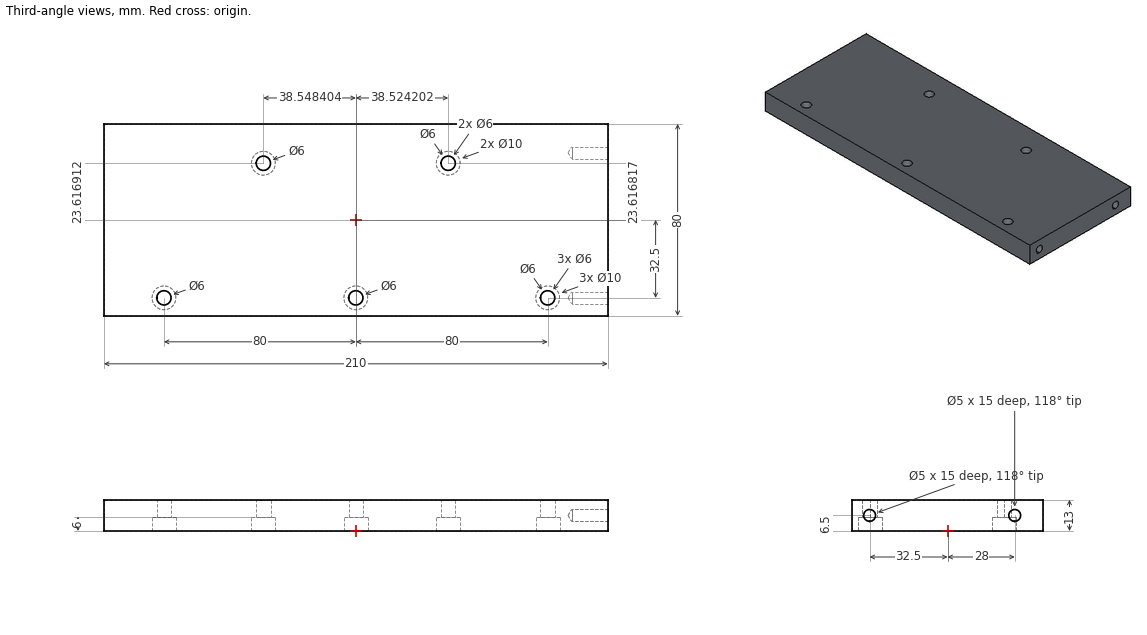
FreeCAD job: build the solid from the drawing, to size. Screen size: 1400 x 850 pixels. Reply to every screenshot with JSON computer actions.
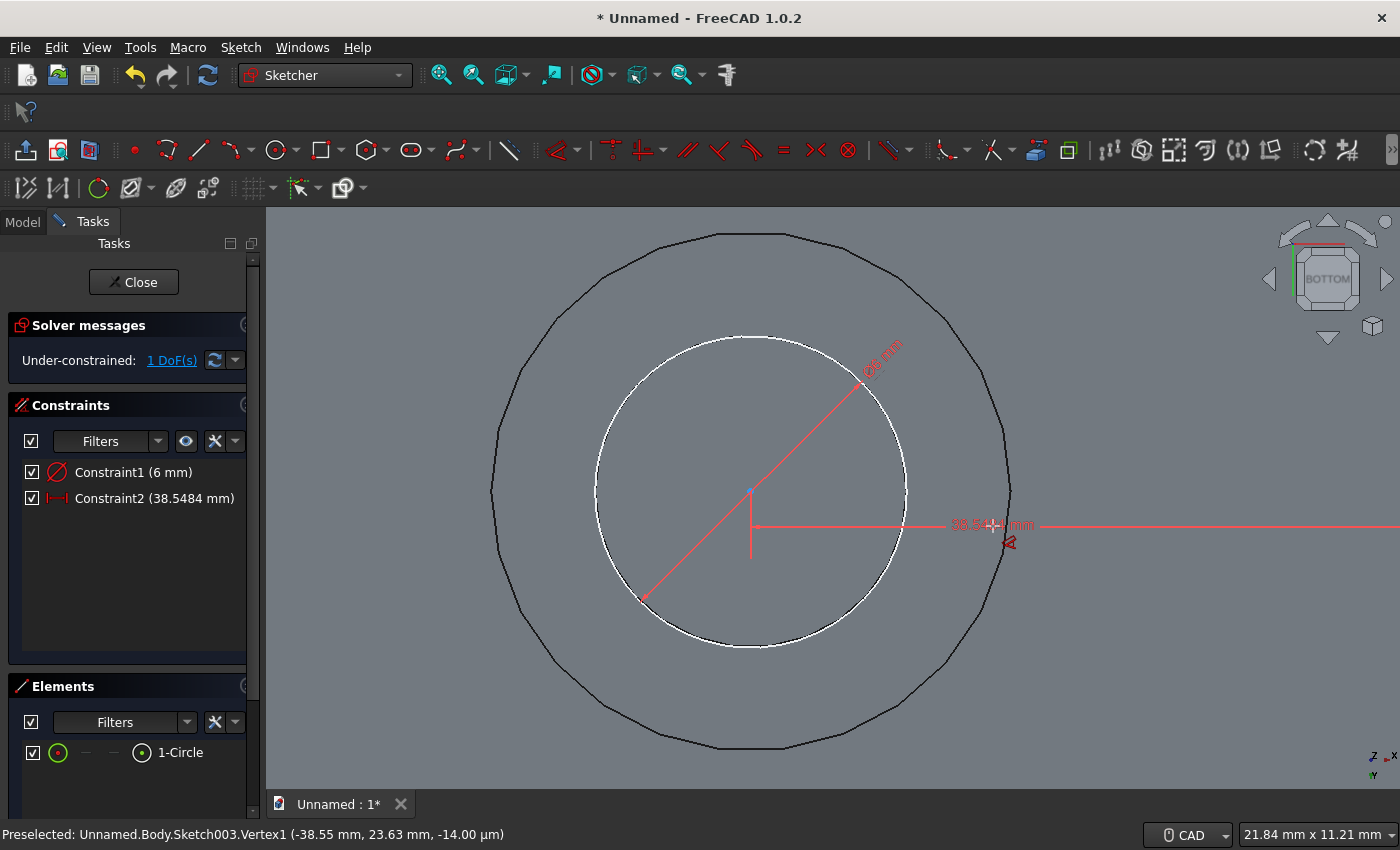
{"action": "left_click", "coordinate": [751, 492]}
{"action": "left_click", "coordinate": [717, 364]}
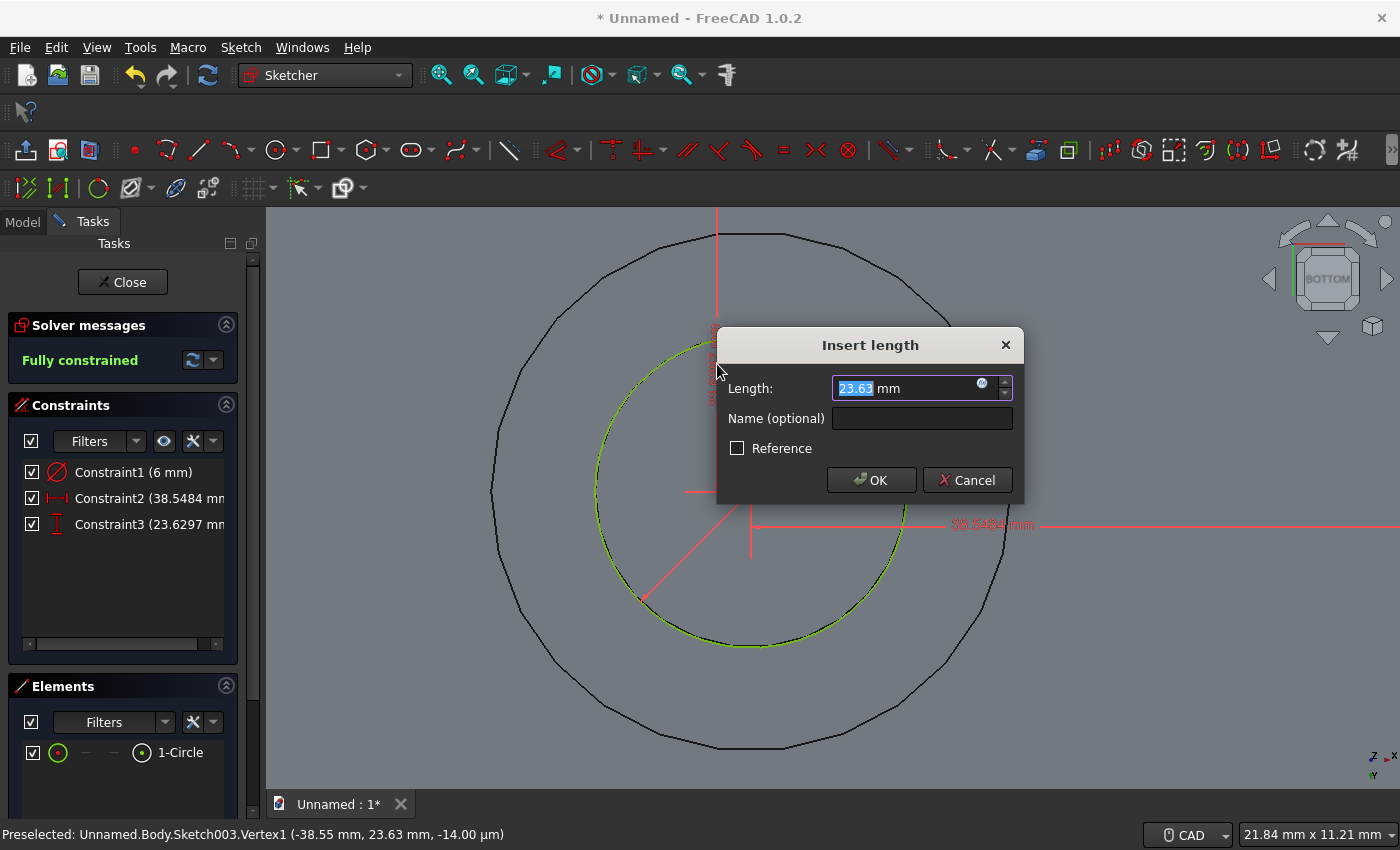
{"action": "type", "text": "23.616912"}
{"action": "key", "text": "Return"}
{"action": "key", "text": "Escape"}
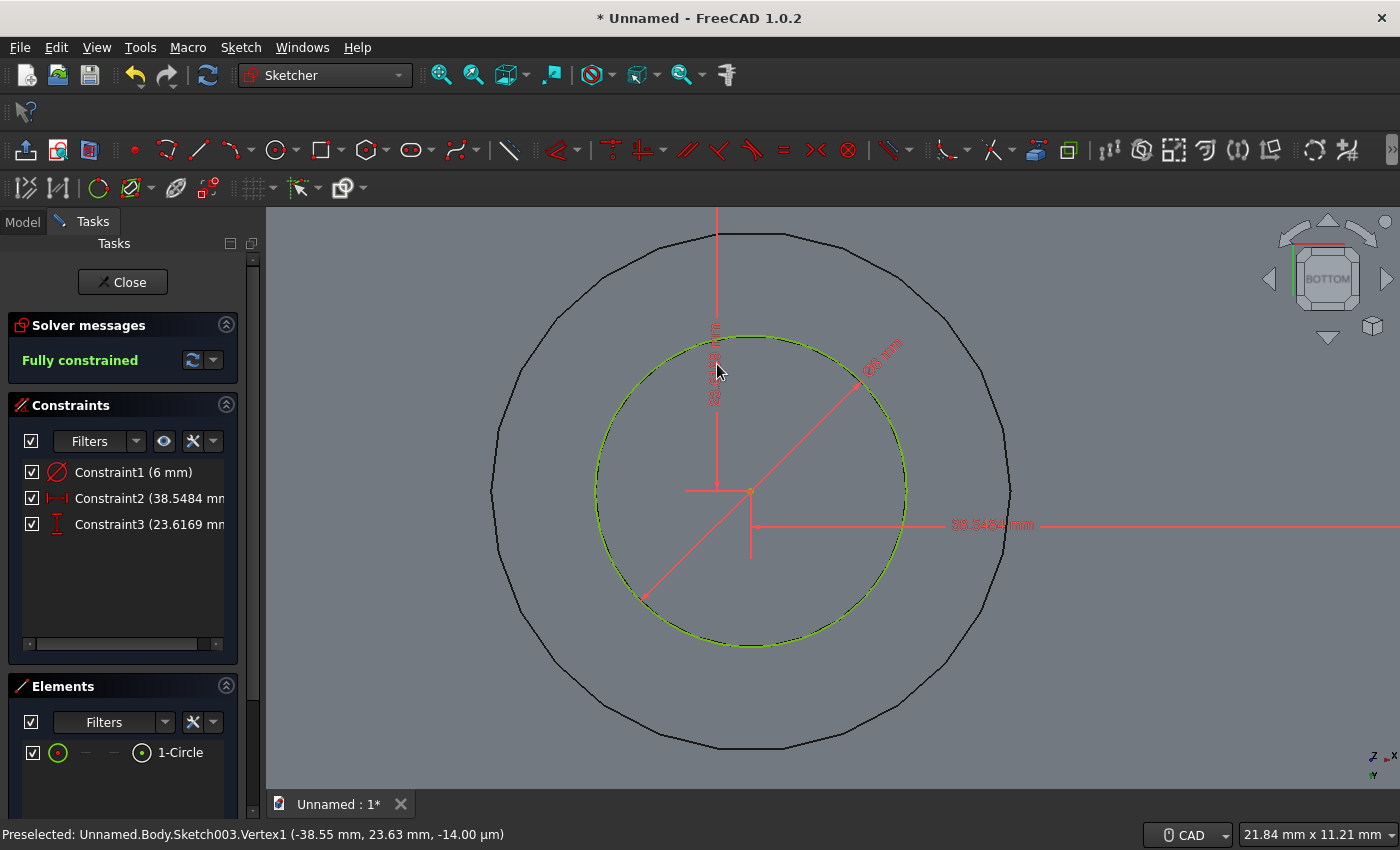
{"action": "left_click", "coordinate": [123, 282]}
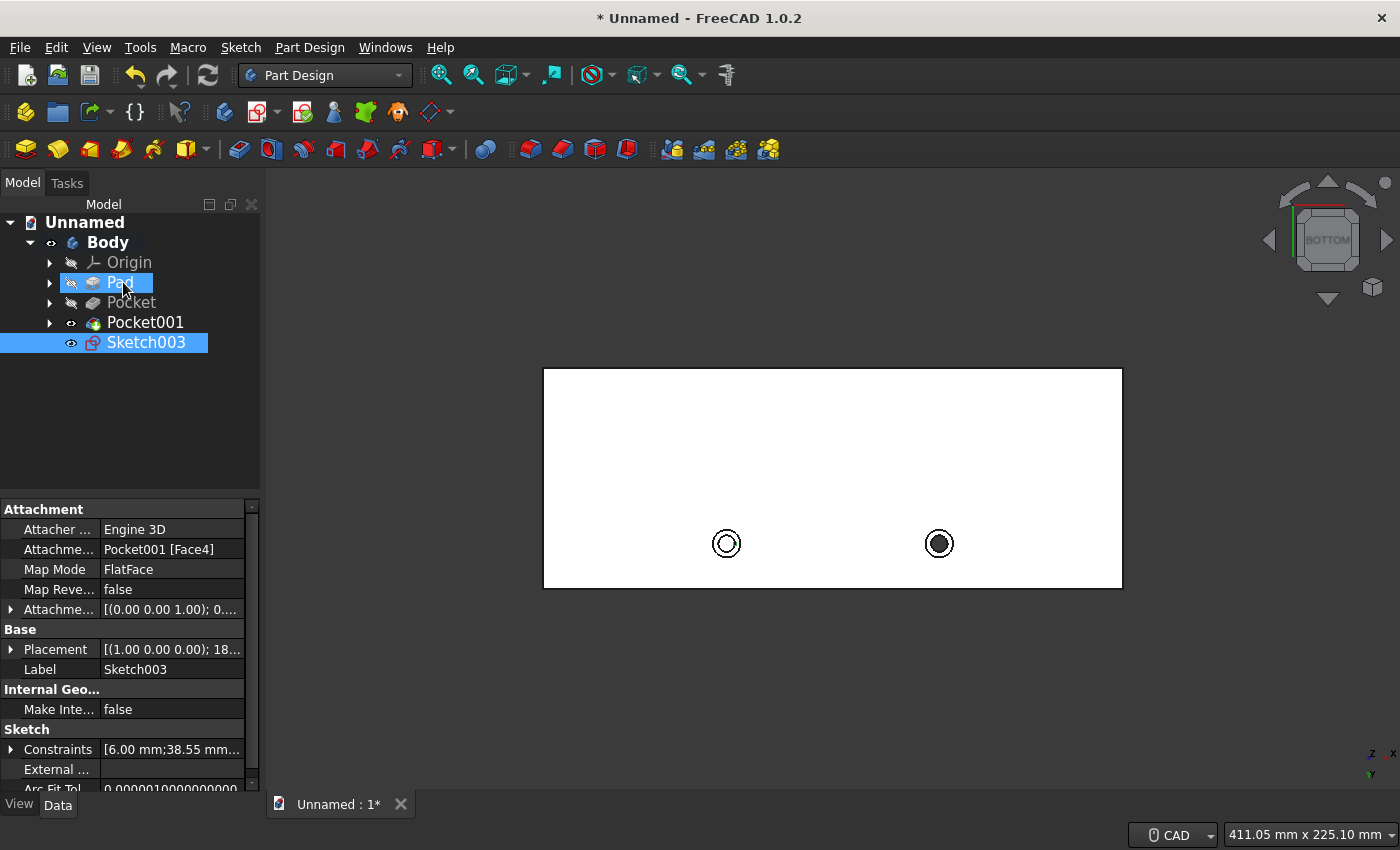
{"action": "left_click", "coordinate": [240, 150]}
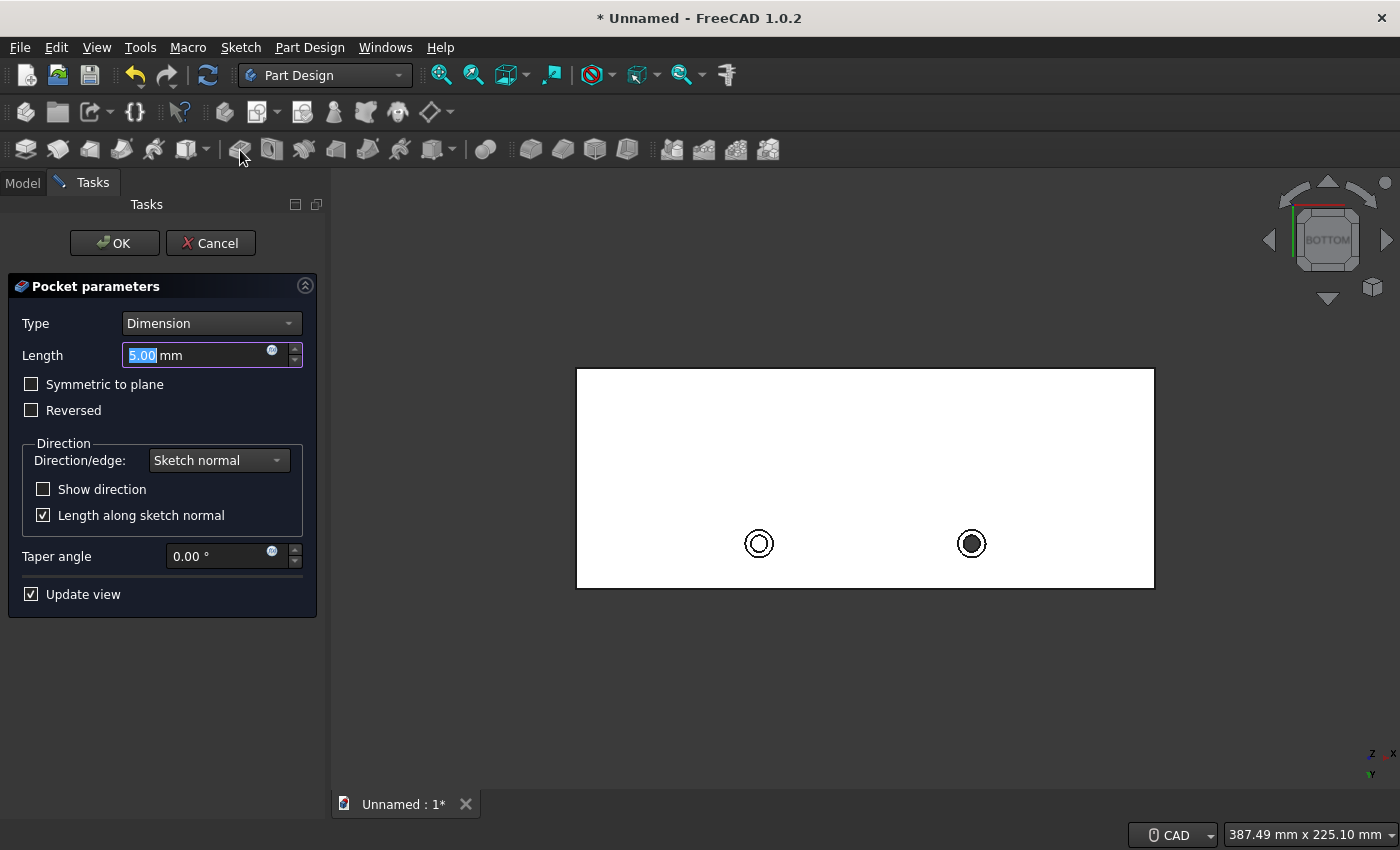
{"action": "left_click", "coordinate": [212, 324]}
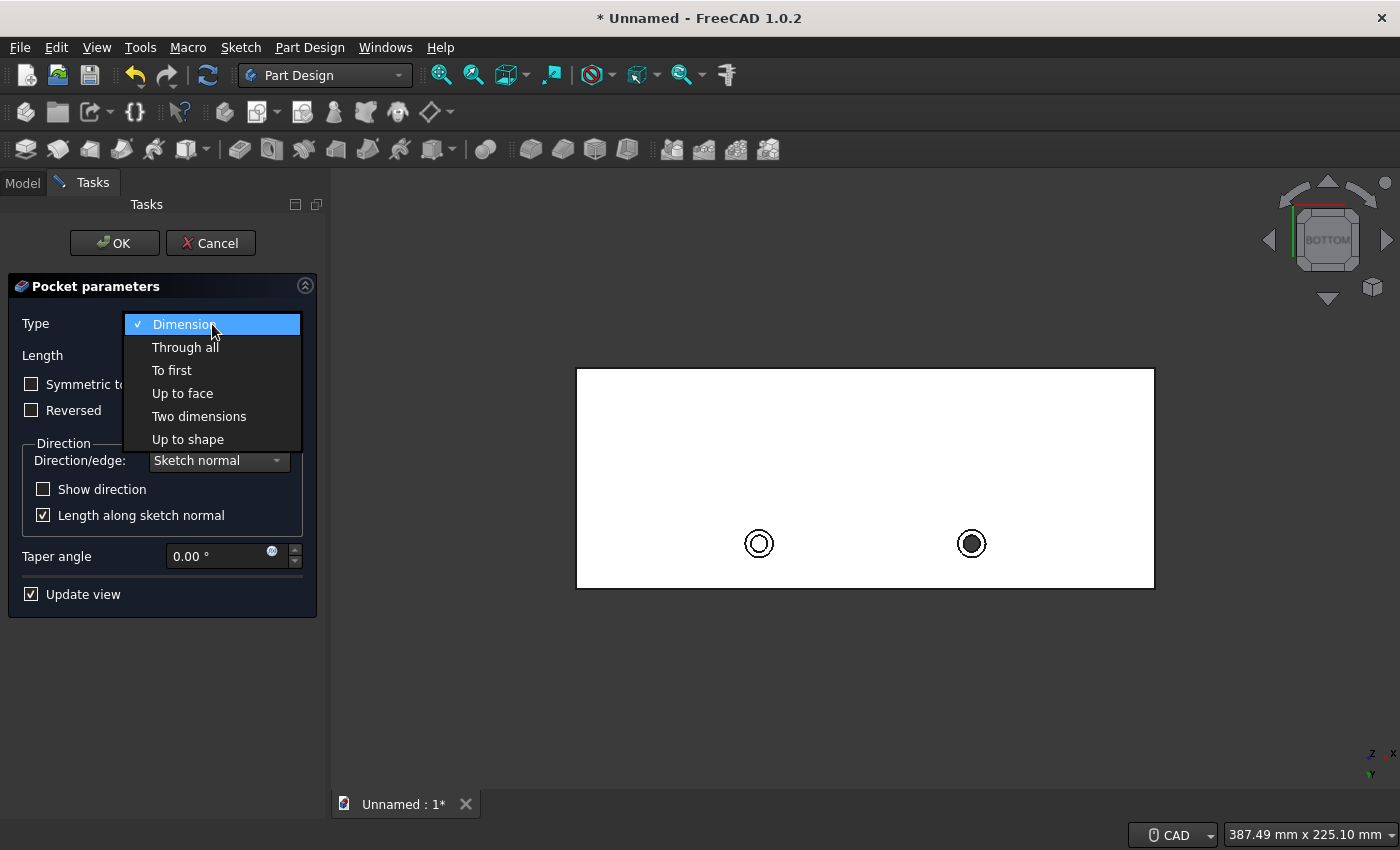
{"action": "left_click", "coordinate": [212, 370]}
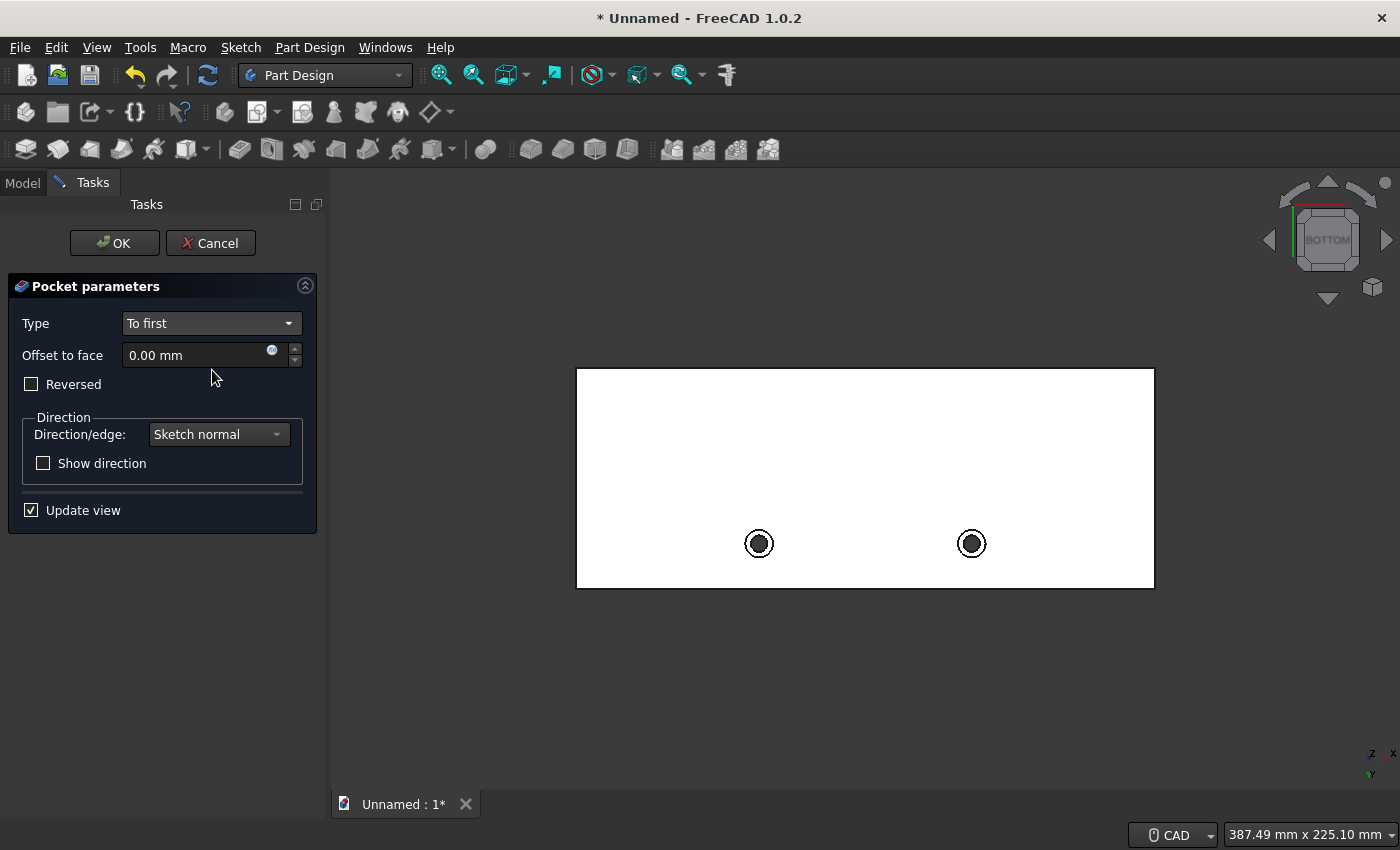
{"action": "left_click", "coordinate": [115, 243]}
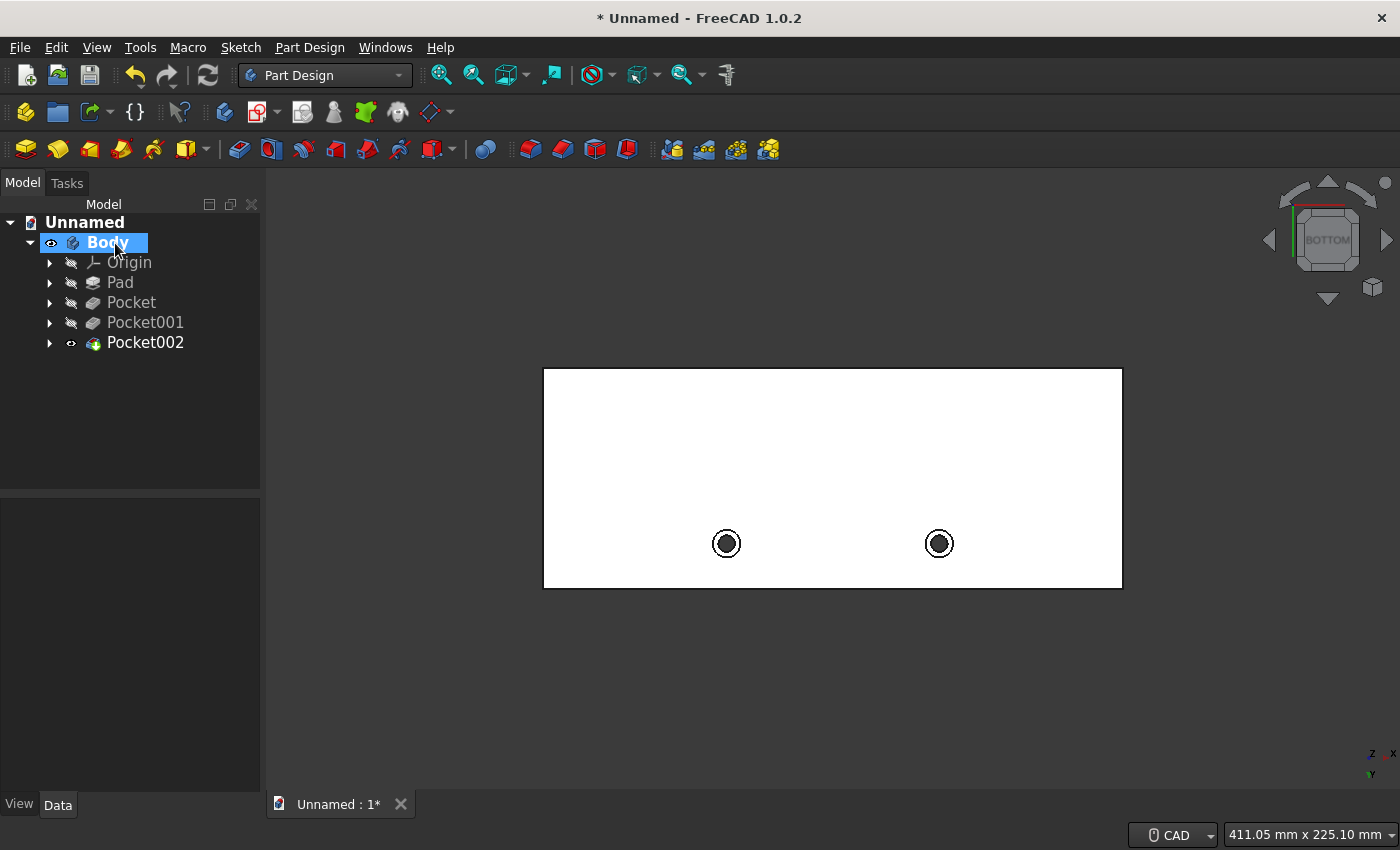
{"action": "key", "text": "0"}